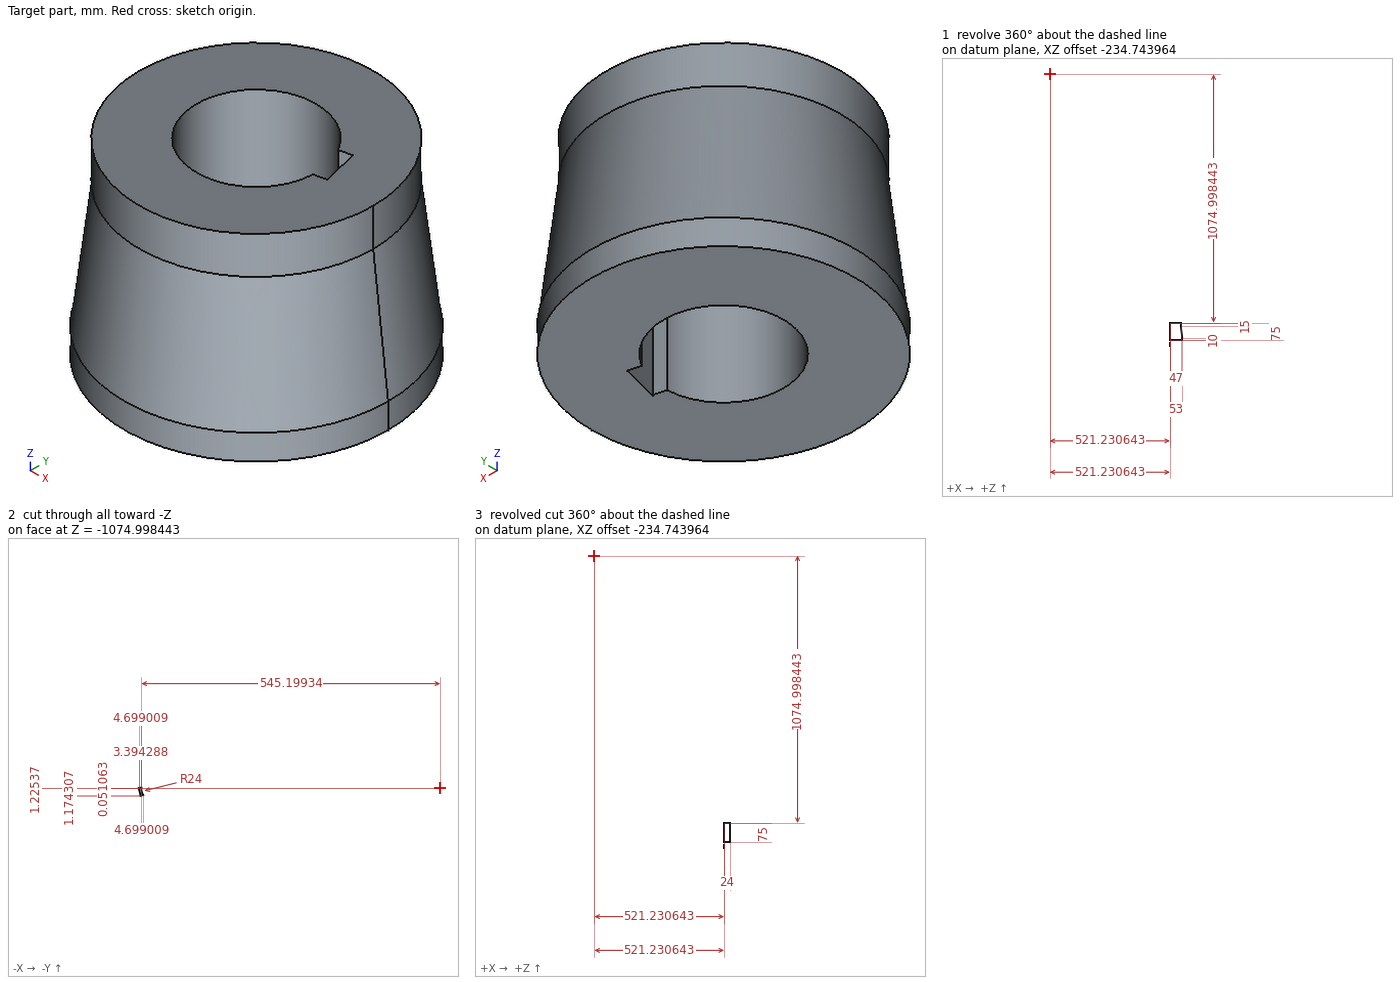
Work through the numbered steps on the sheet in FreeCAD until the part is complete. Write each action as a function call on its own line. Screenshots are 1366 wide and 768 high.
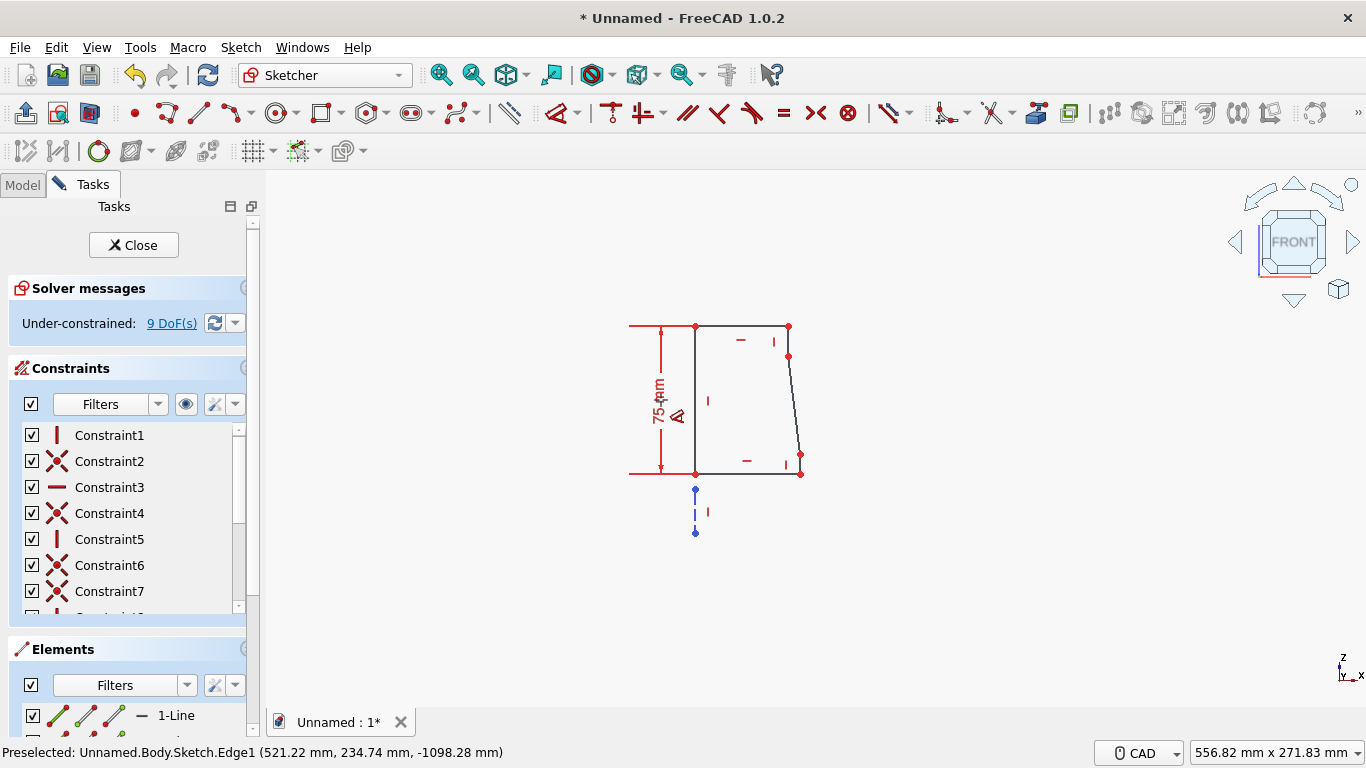
click(726, 474)
click(747, 508)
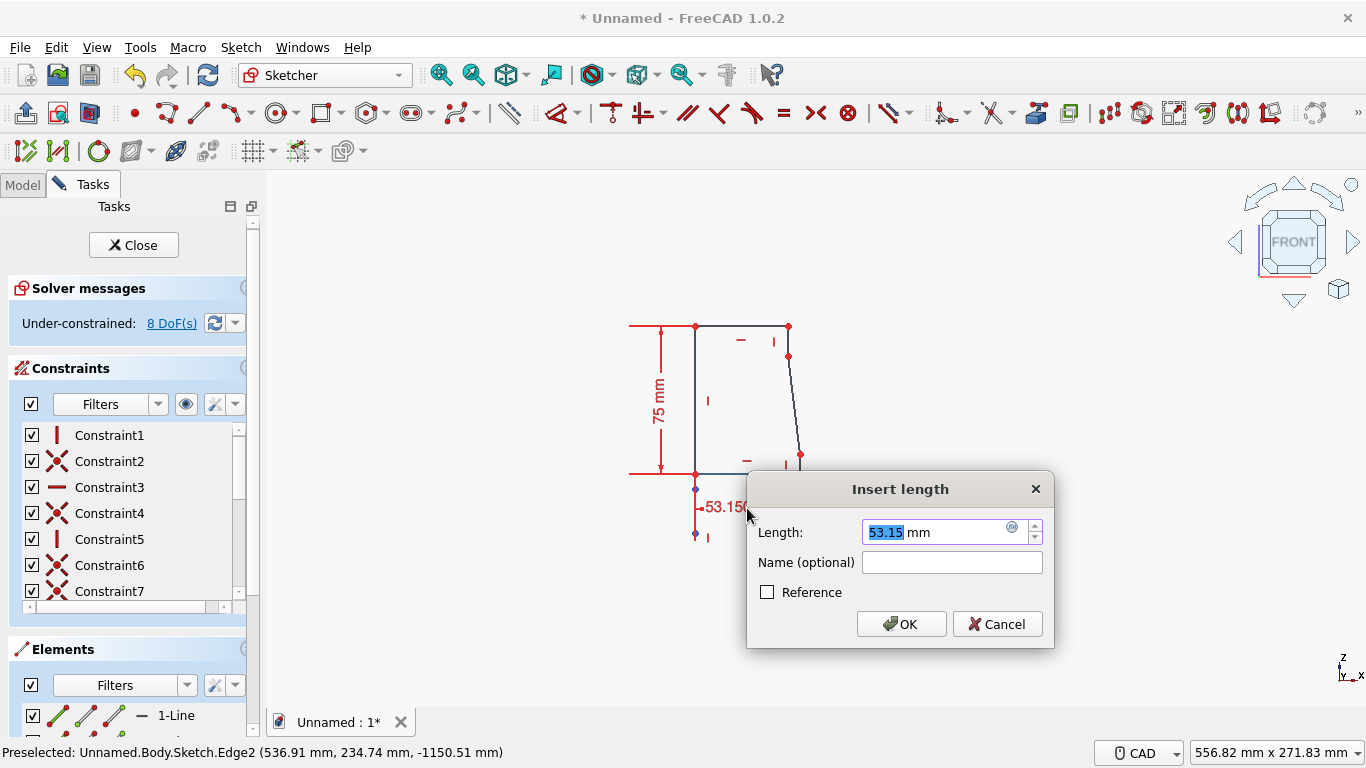
text(53)
key(Return)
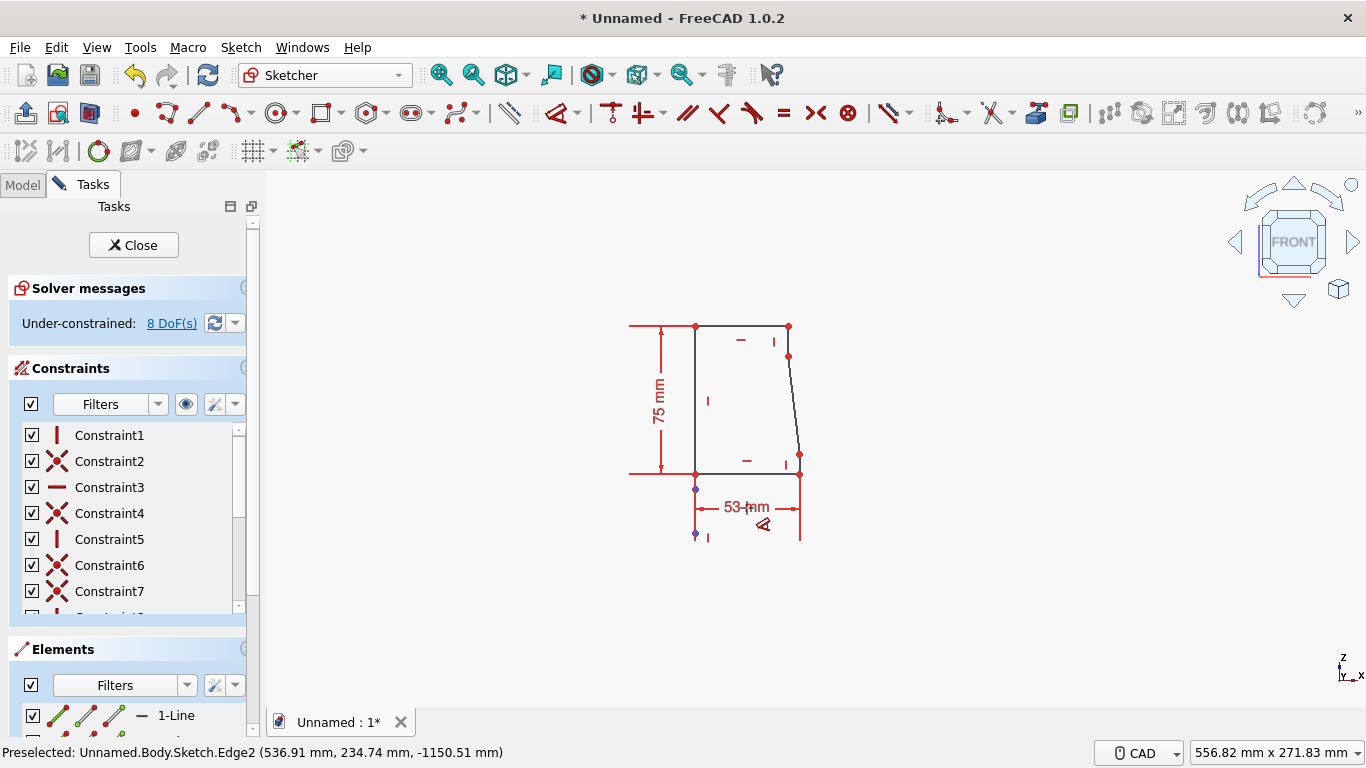
scroll(800, 464, up, 4)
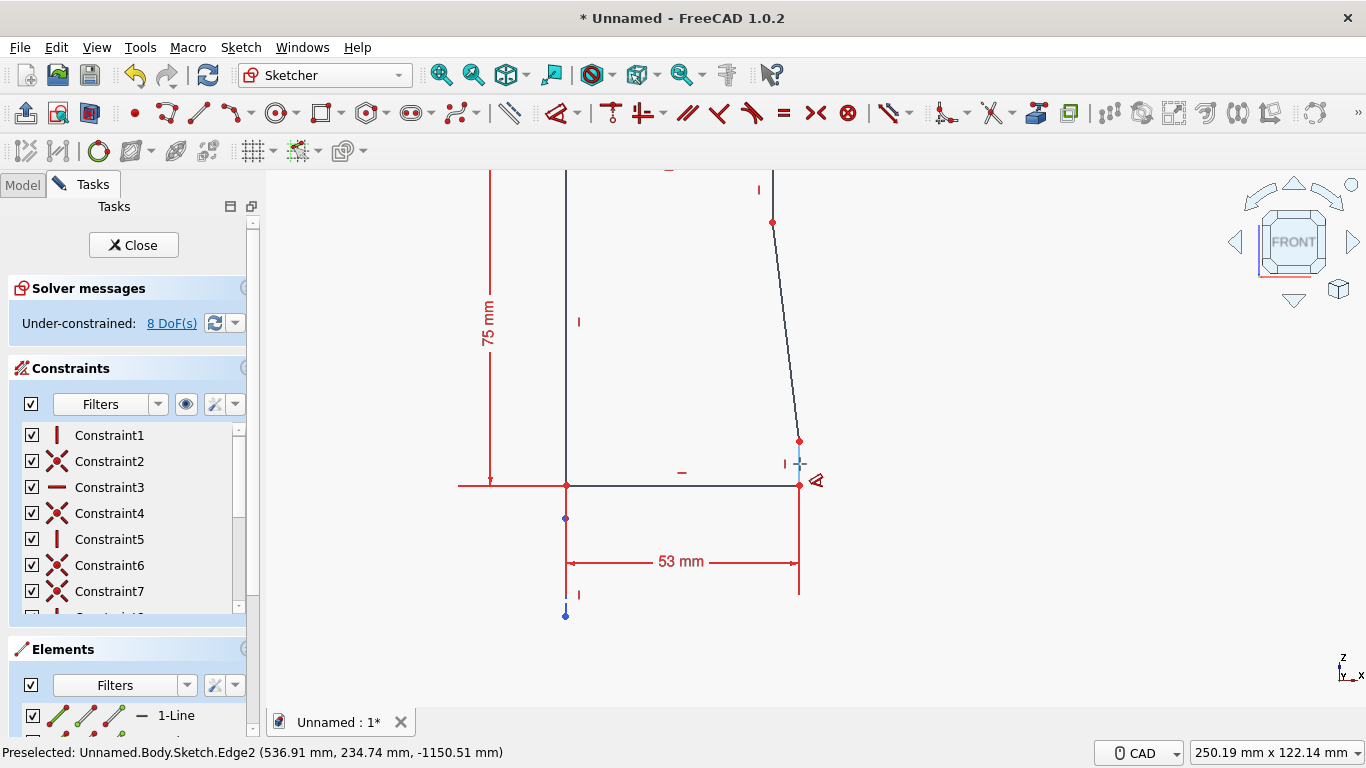
click(799, 464)
click(833, 464)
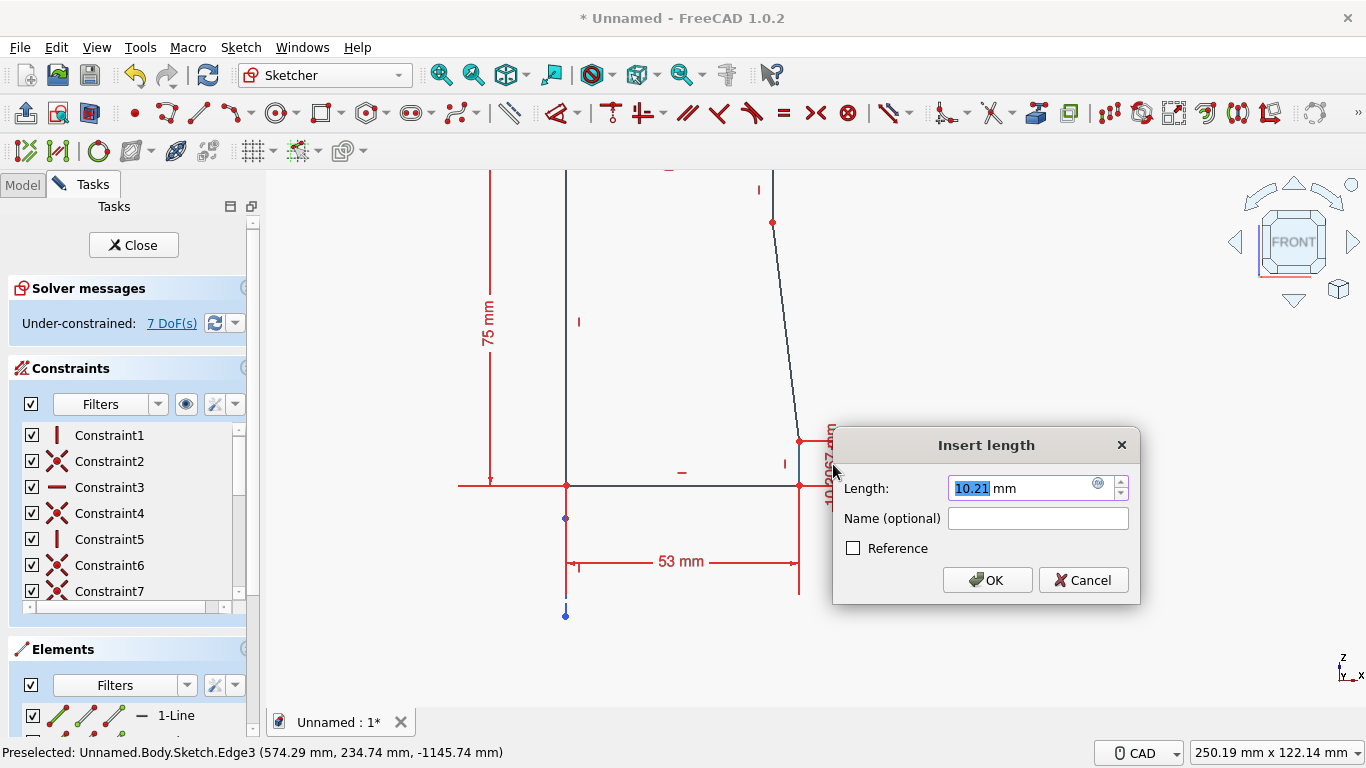
text(10)
key(Return)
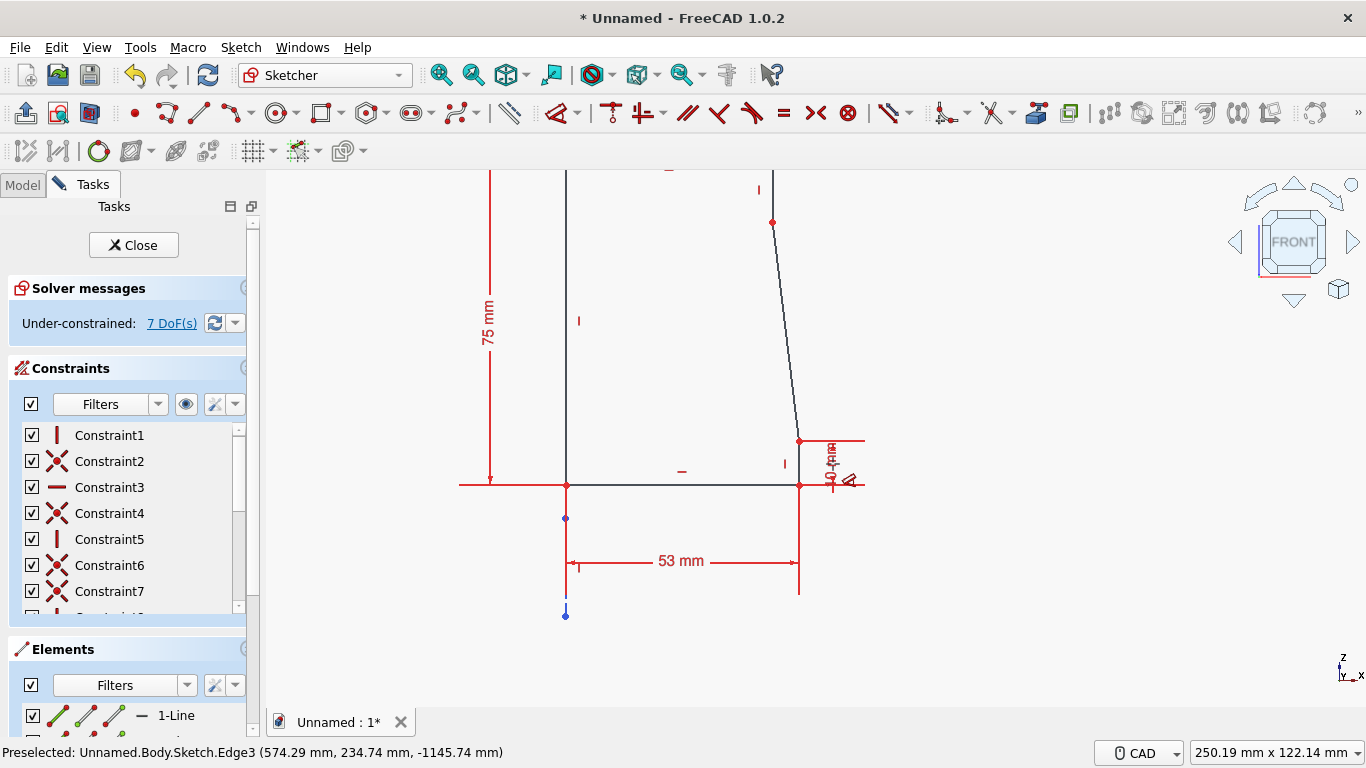
click(773, 203)
click(807, 210)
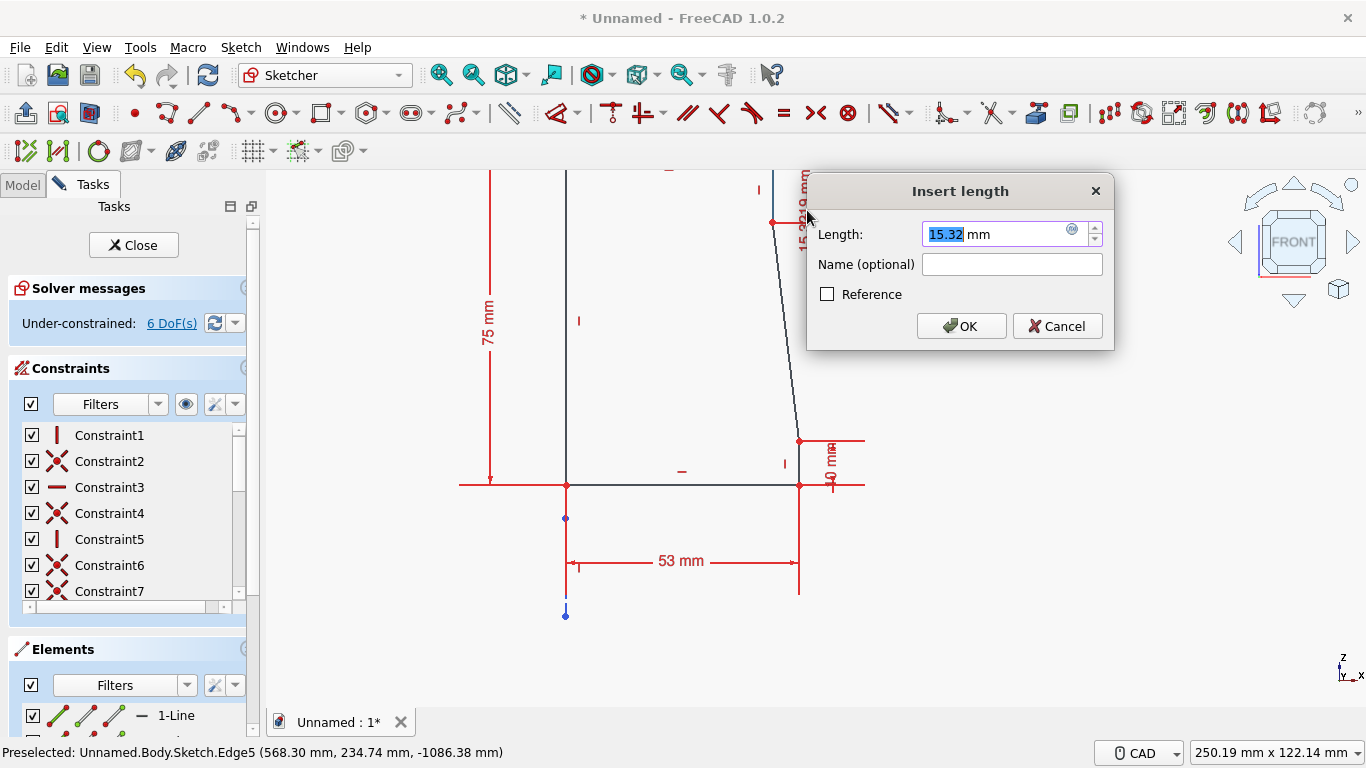
text(15)
key(Return)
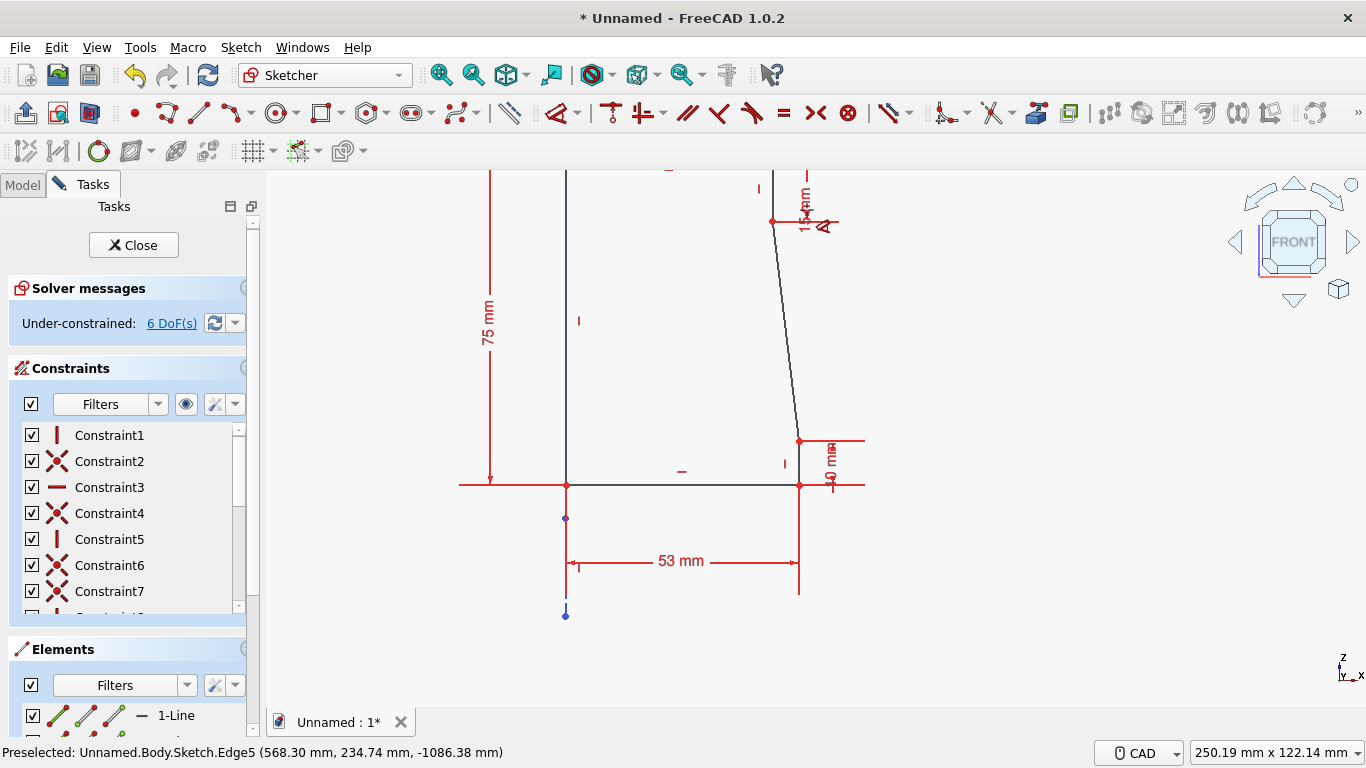
scroll(880, 548, down, 2)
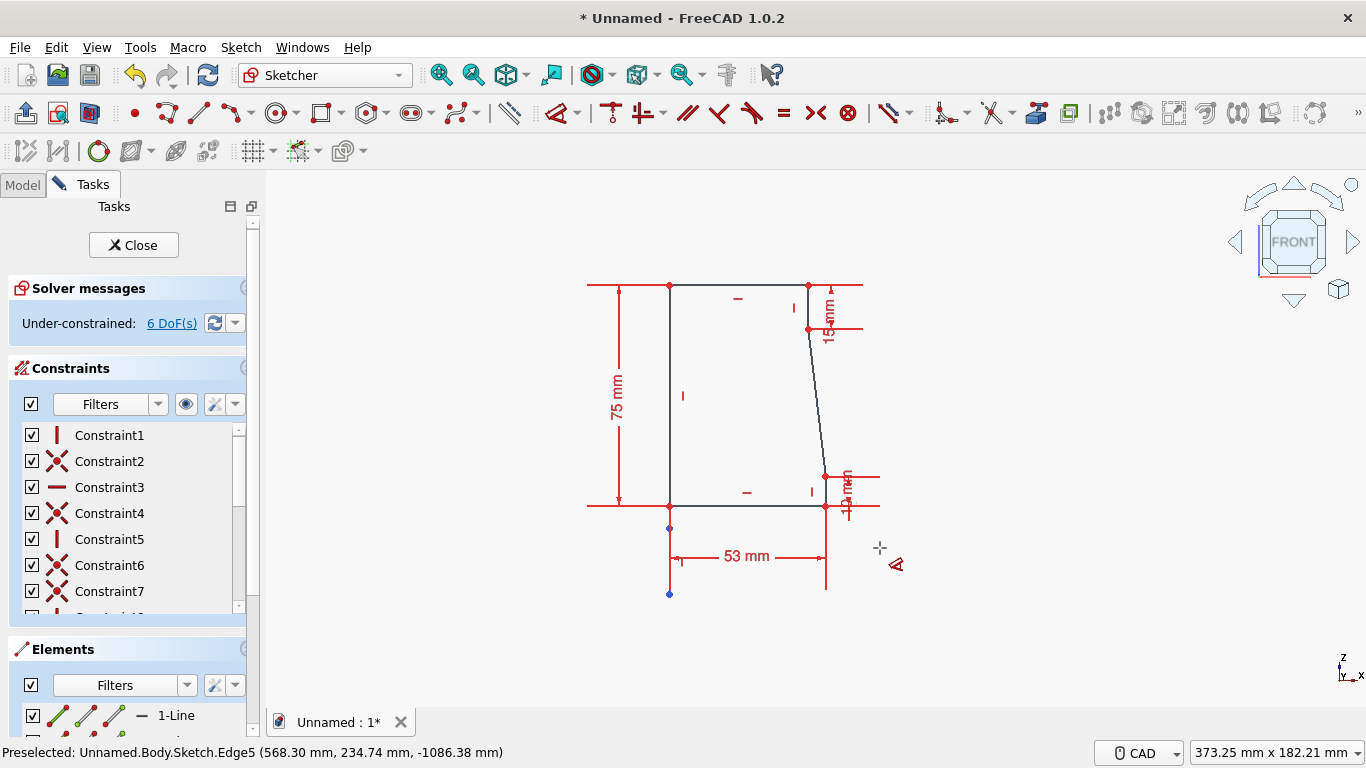
click(767, 285)
click(739, 251)